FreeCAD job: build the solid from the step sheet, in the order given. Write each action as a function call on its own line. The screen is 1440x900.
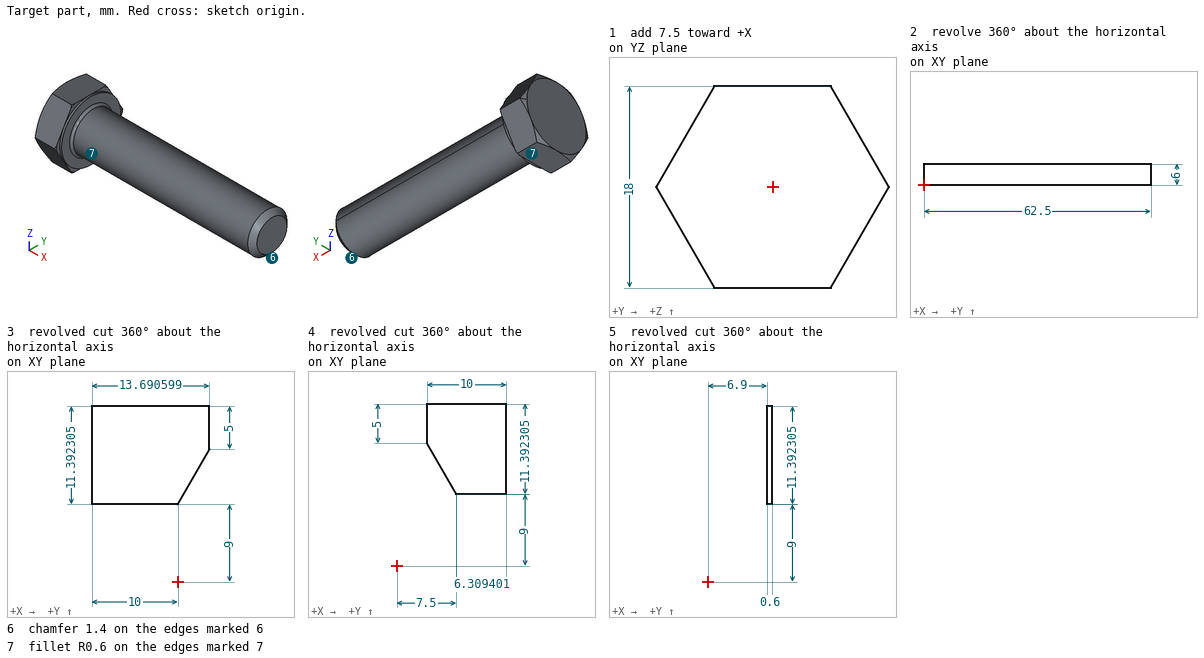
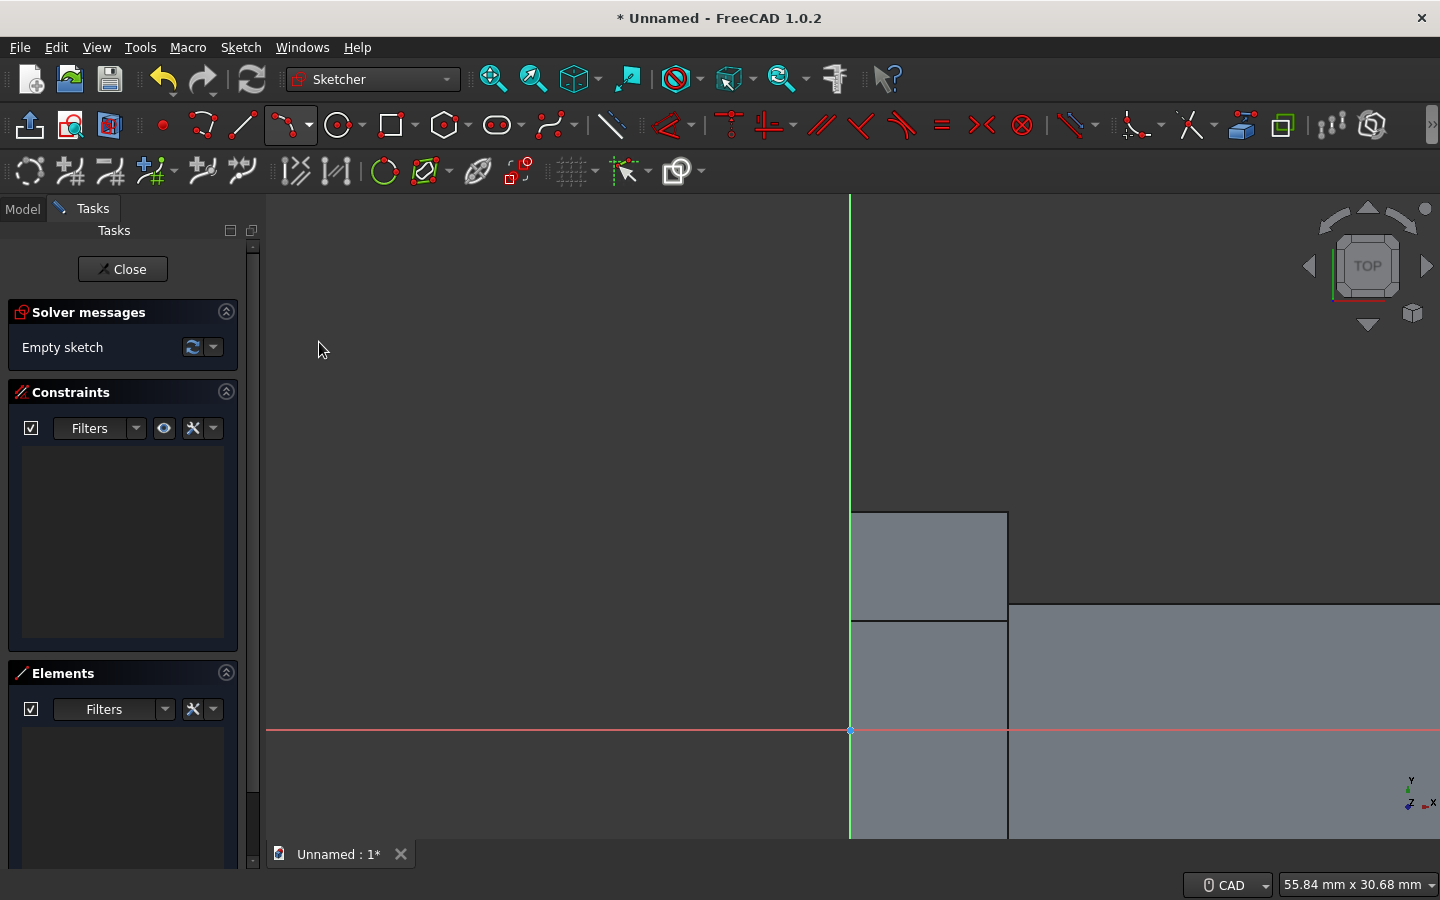
key(g)
key(m)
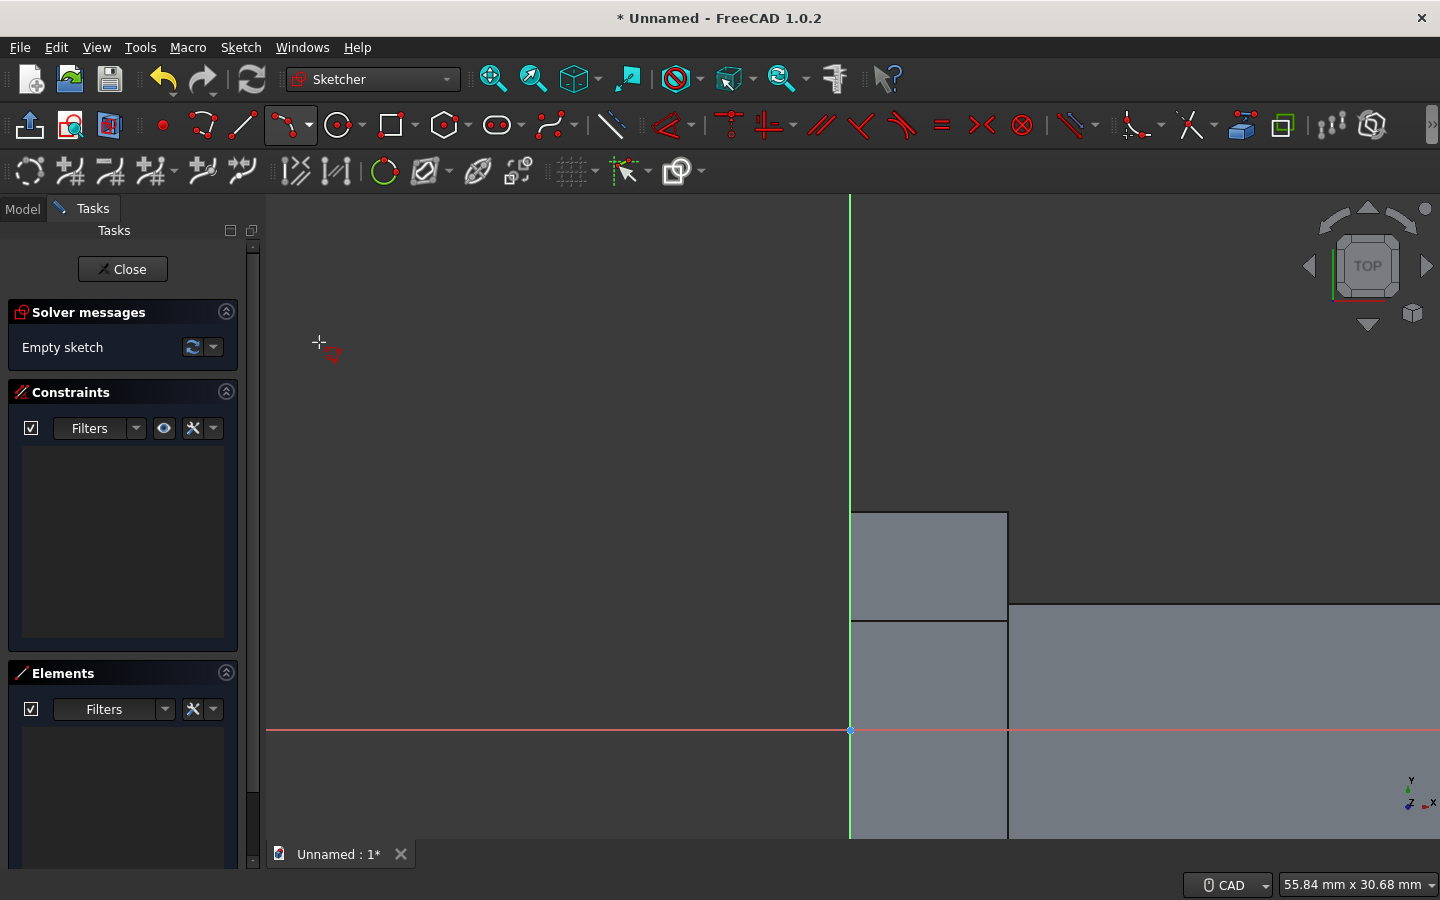
click(850, 541)
click(928, 406)
click(928, 301)
click(640, 301)
click(640, 541)
click(850, 542)
key(Escape)
key(Escape)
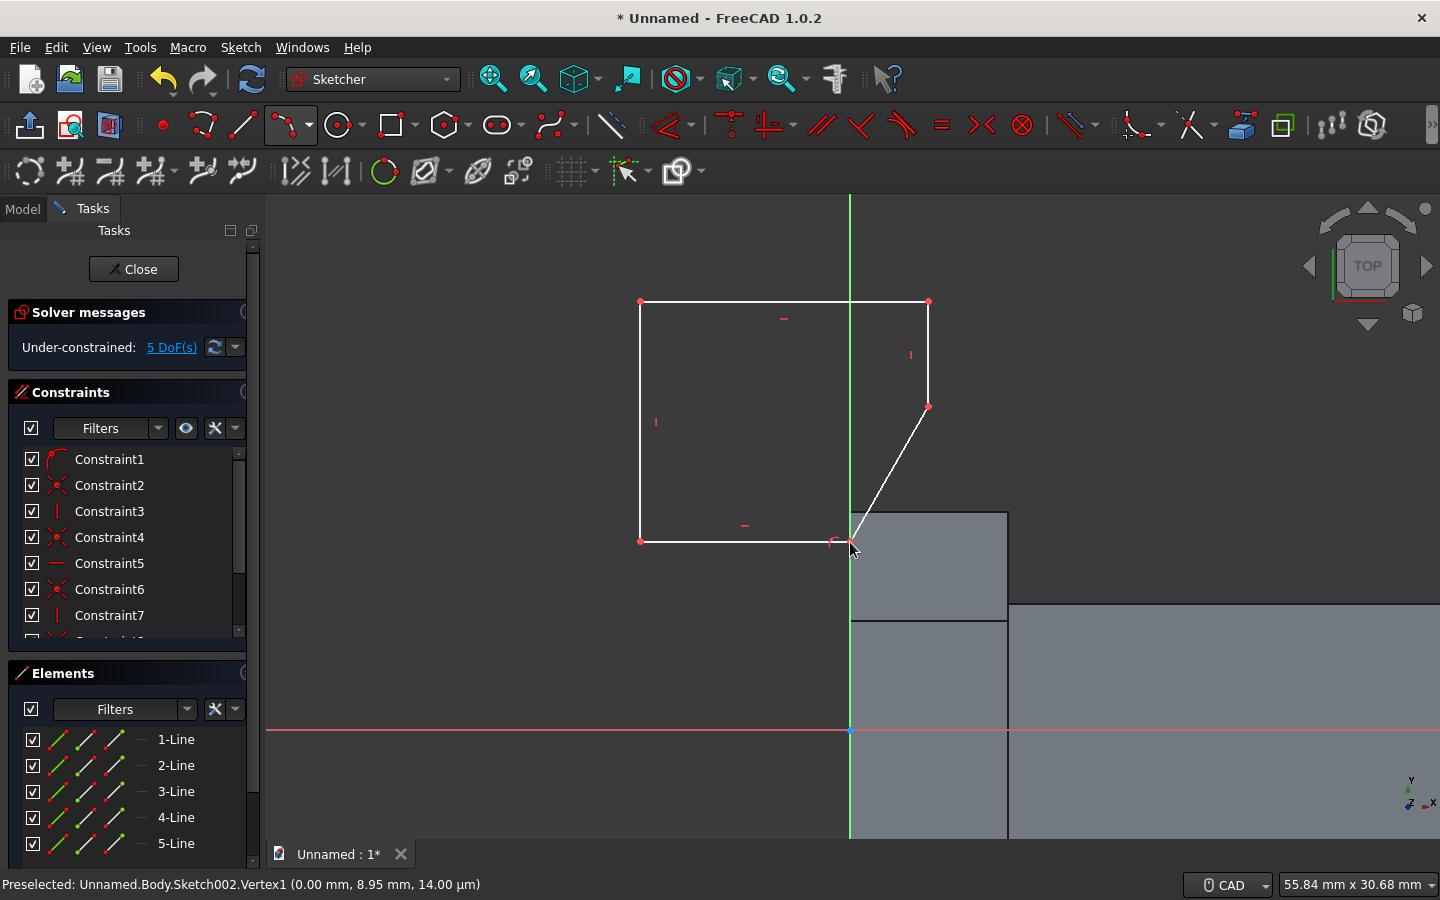
click(666, 126)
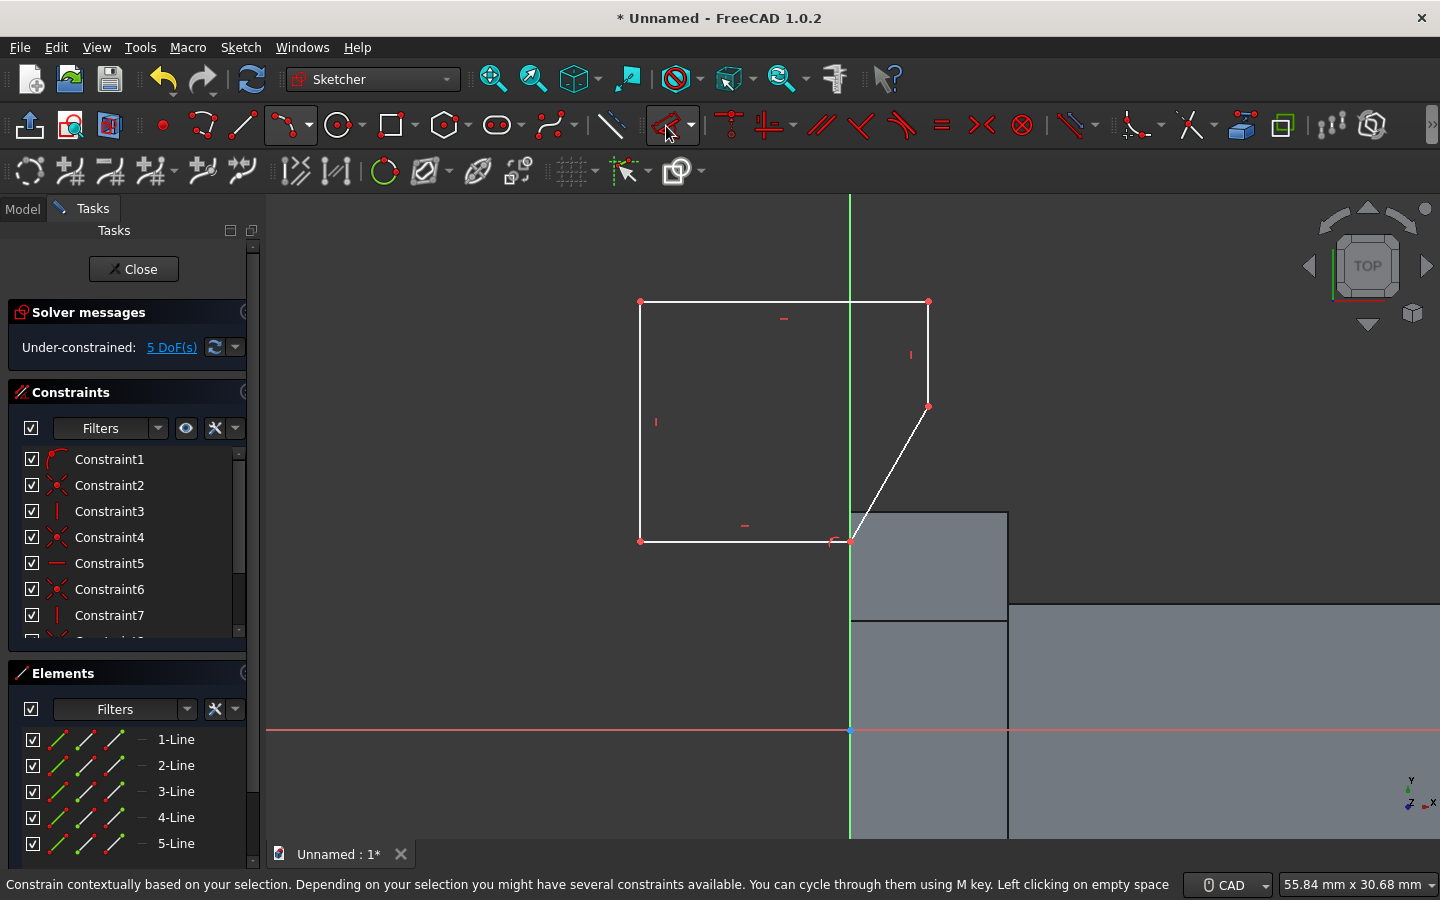
click(928, 375)
click(962, 354)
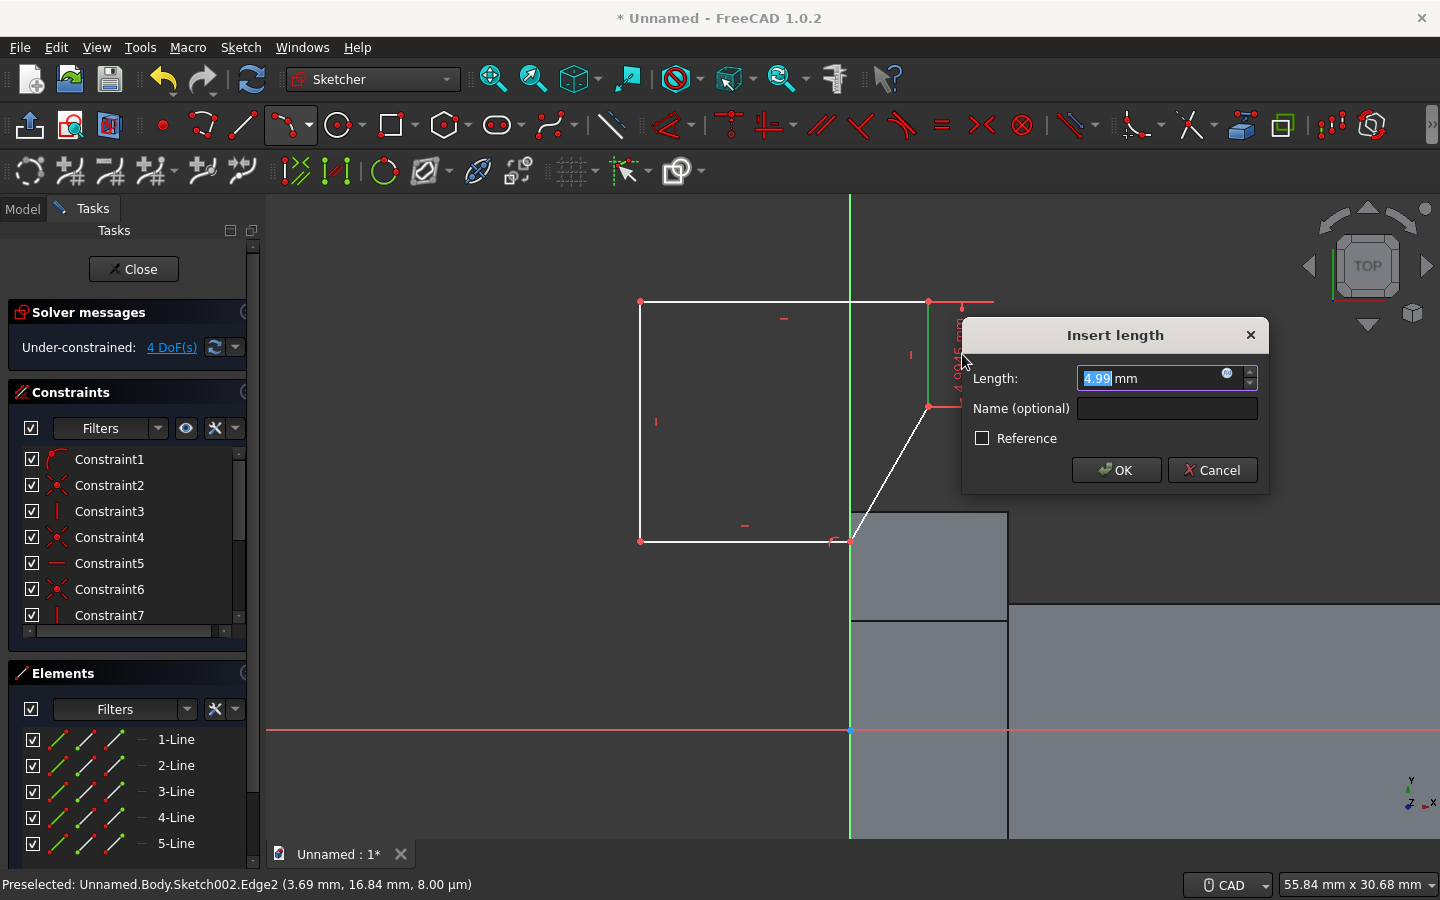
text(5)
key(Return)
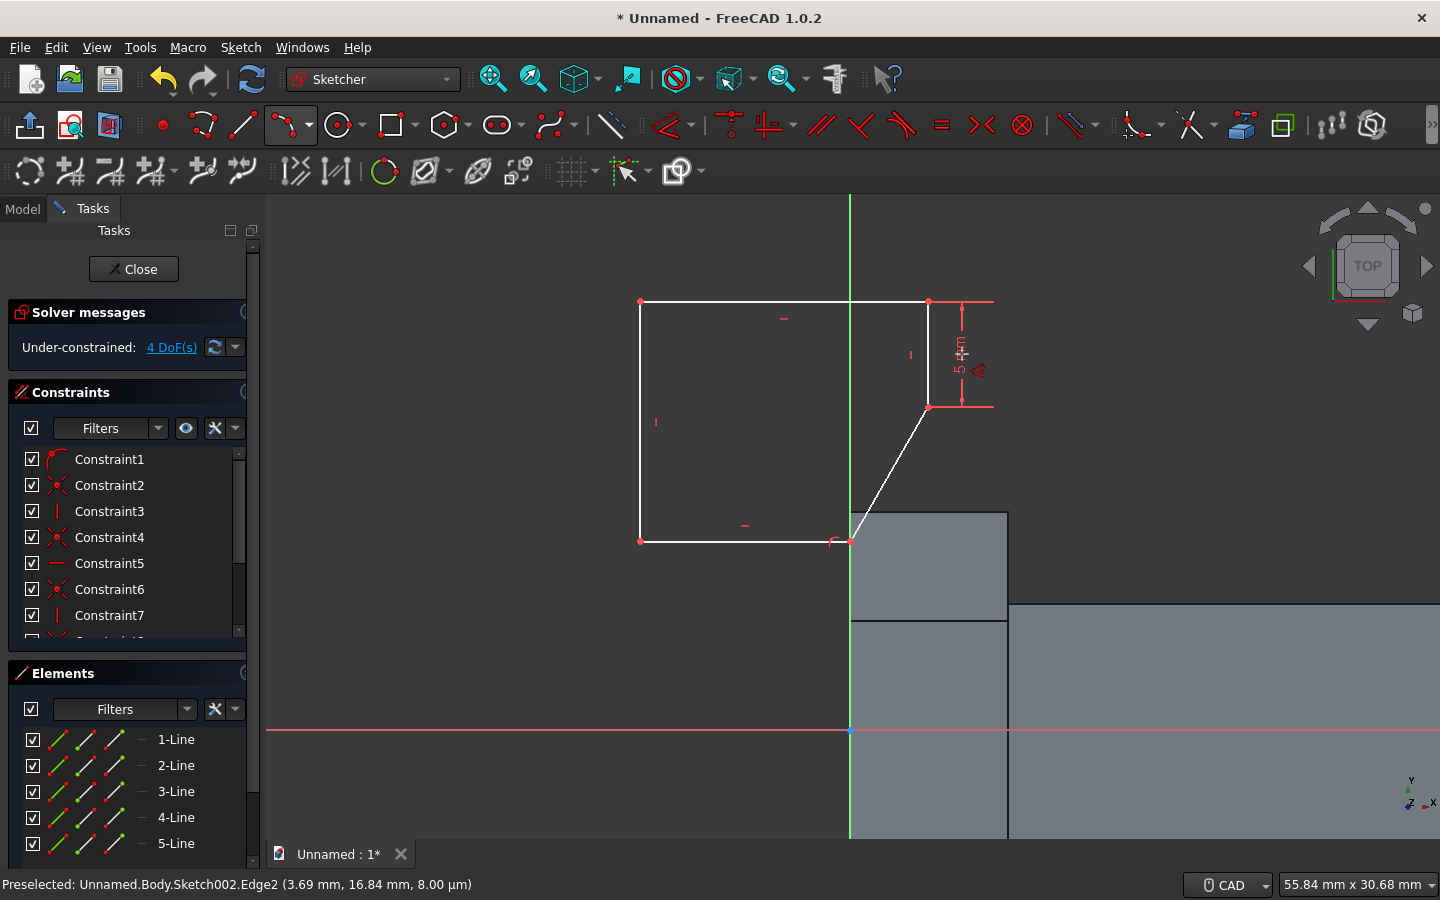
click(703, 542)
click(745, 576)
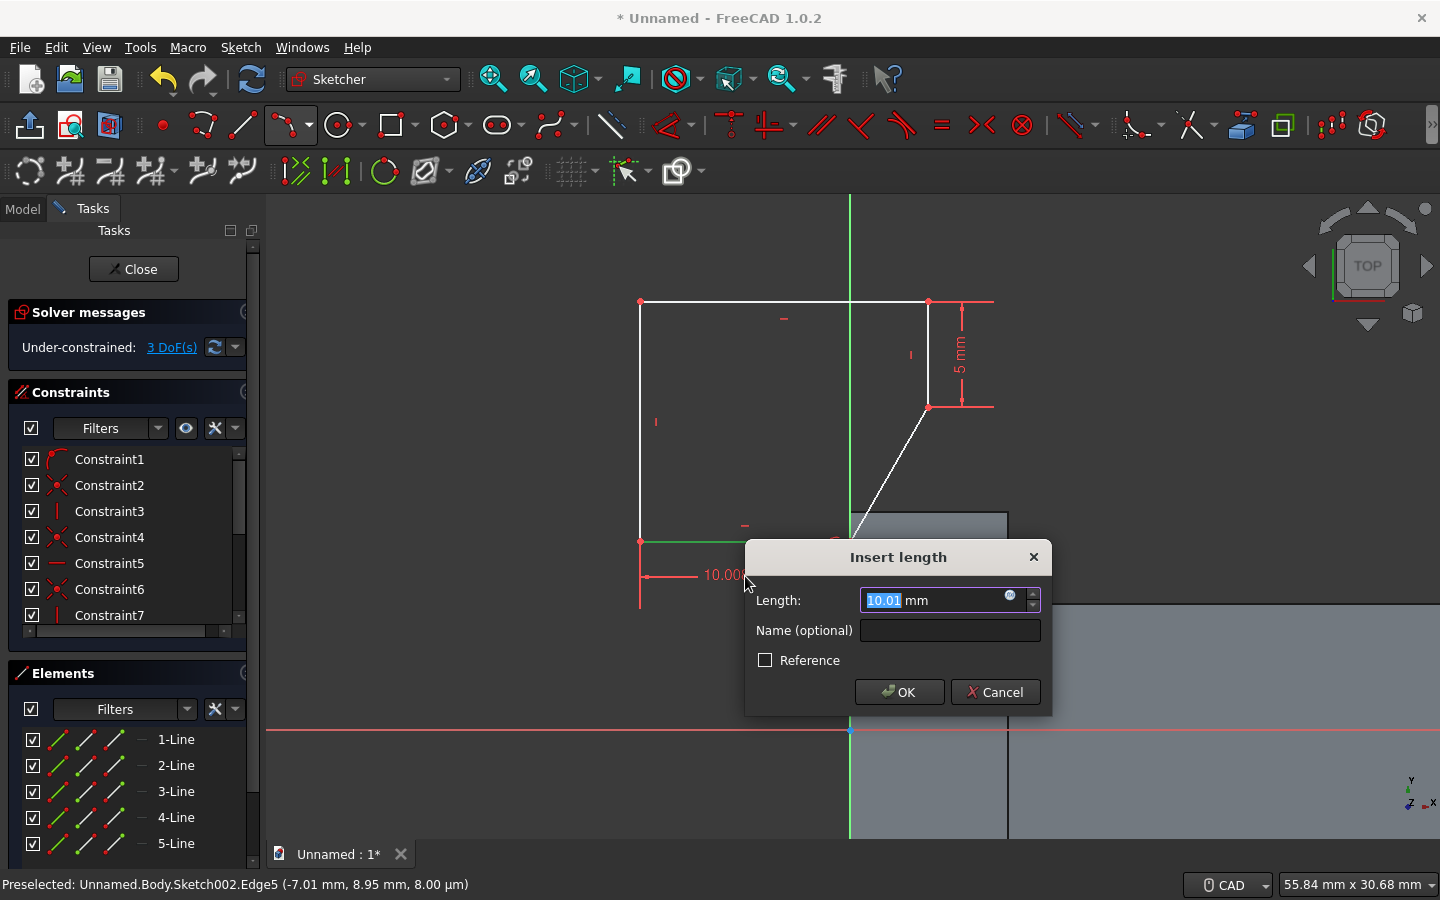
text(10)
key(Return)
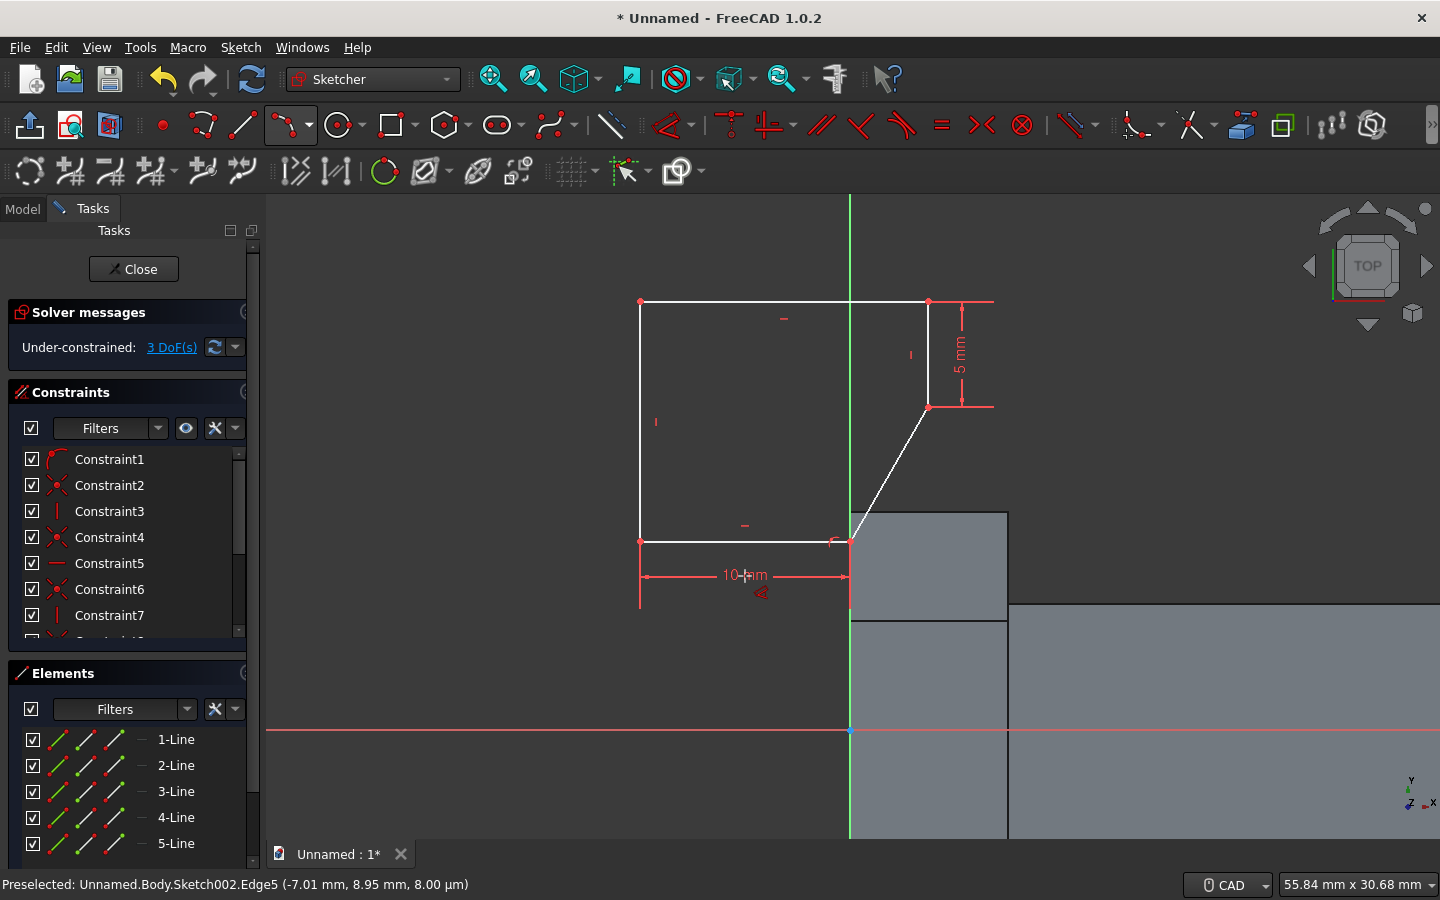
click(850, 542)
click(884, 636)